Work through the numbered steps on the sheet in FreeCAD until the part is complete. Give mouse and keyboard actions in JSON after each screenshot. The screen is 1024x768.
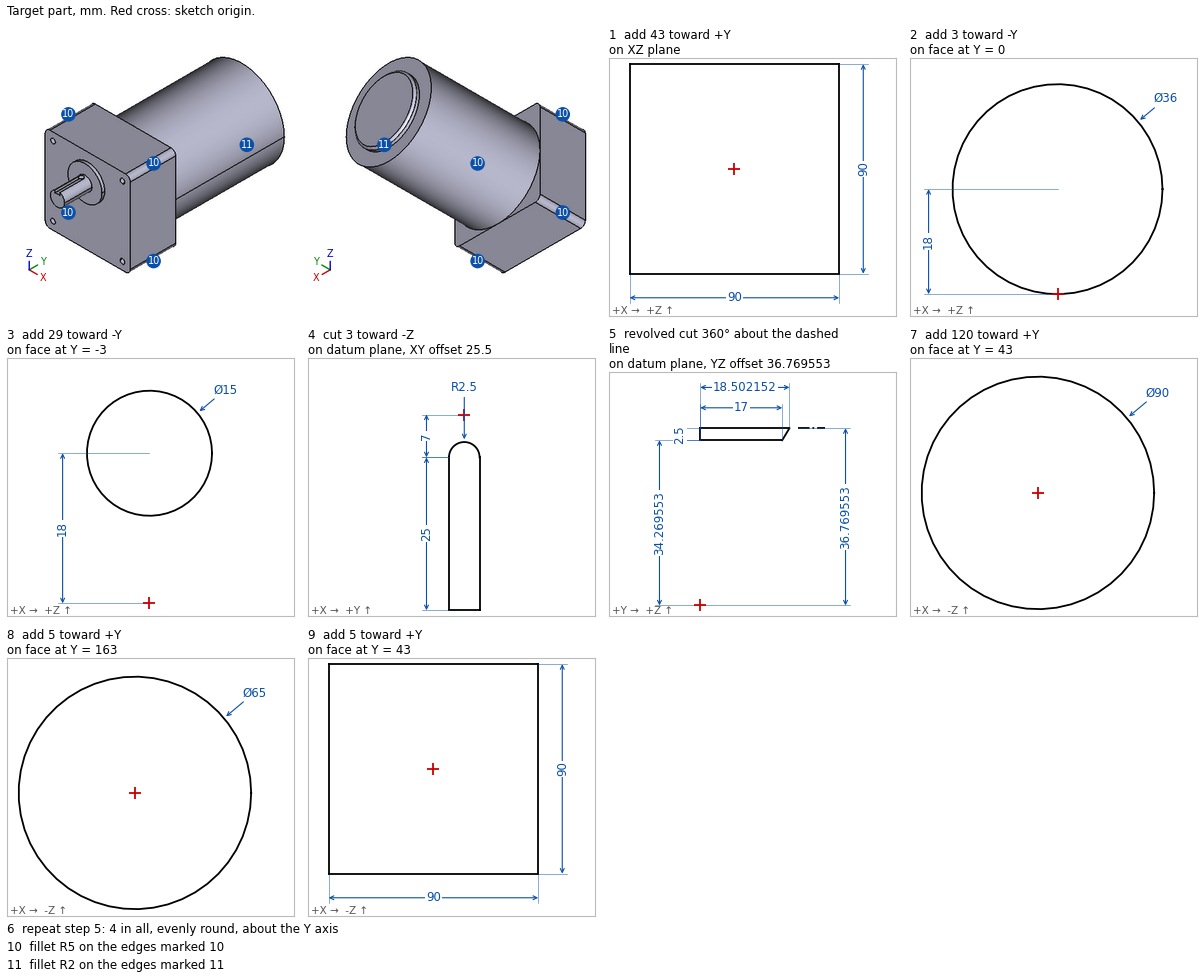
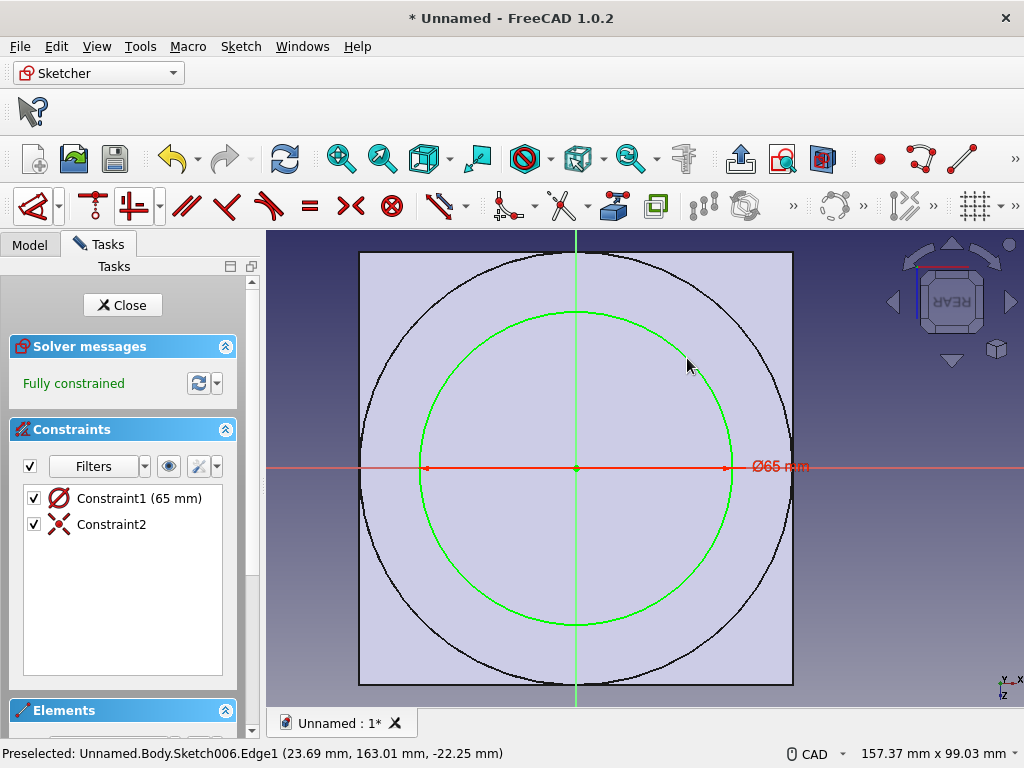
{"action": "left_click", "coordinate": [123, 305]}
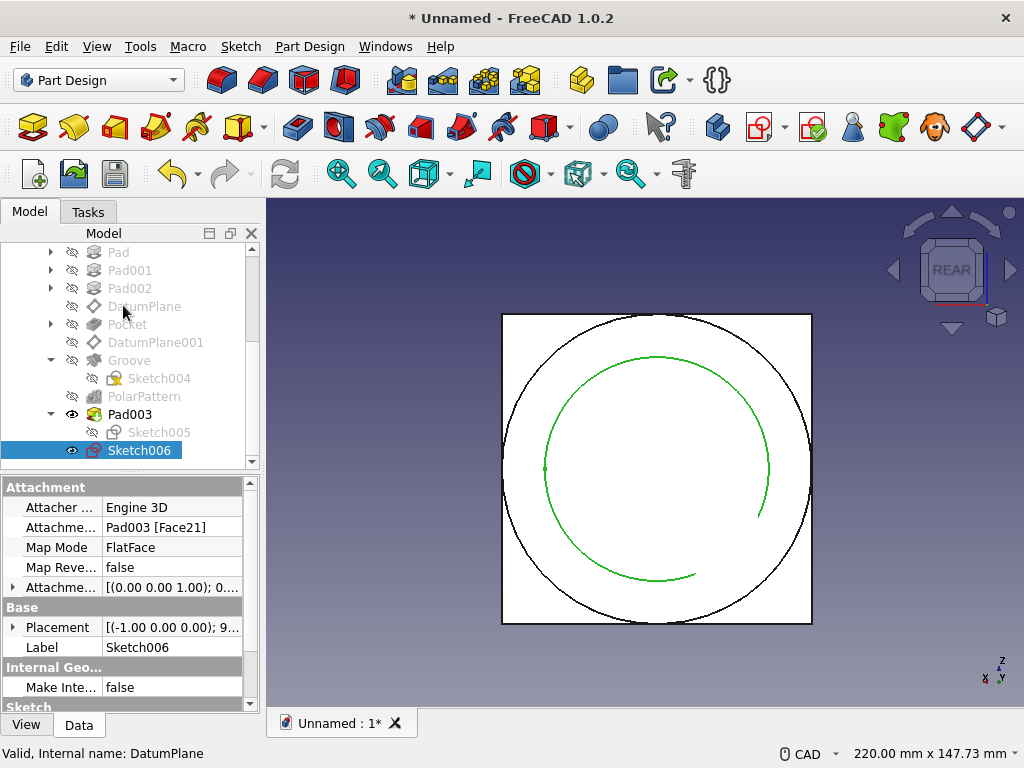
{"action": "left_click", "coordinate": [33, 128]}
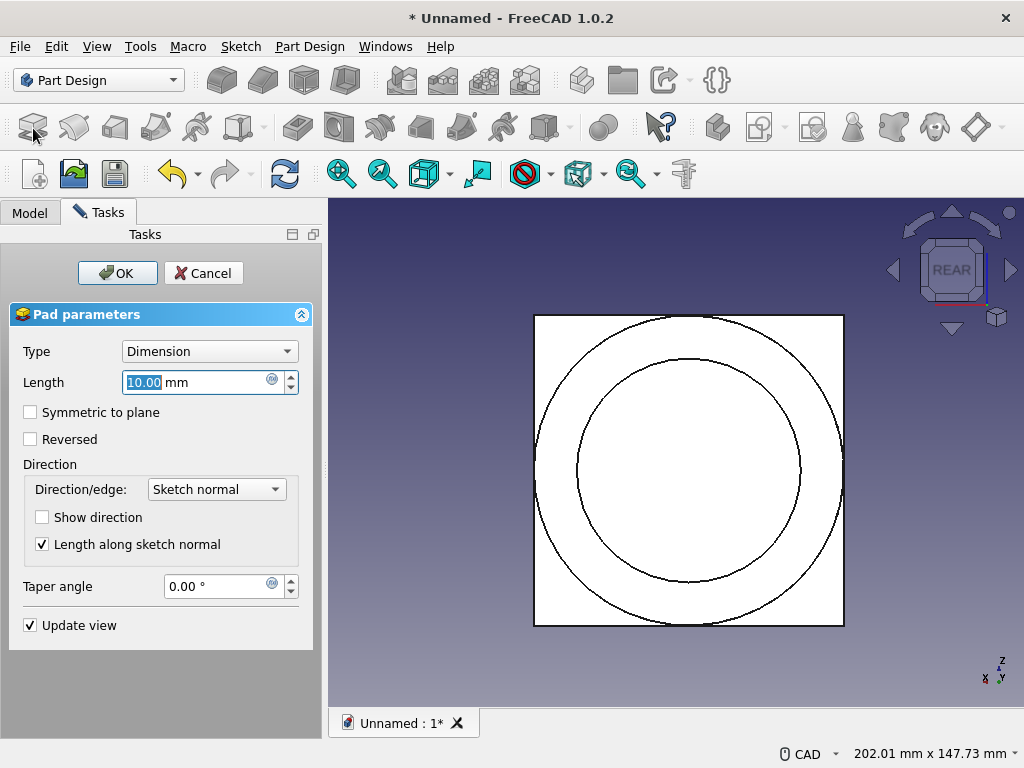
{"action": "type", "text": "5"}
{"action": "key", "text": "Tab"}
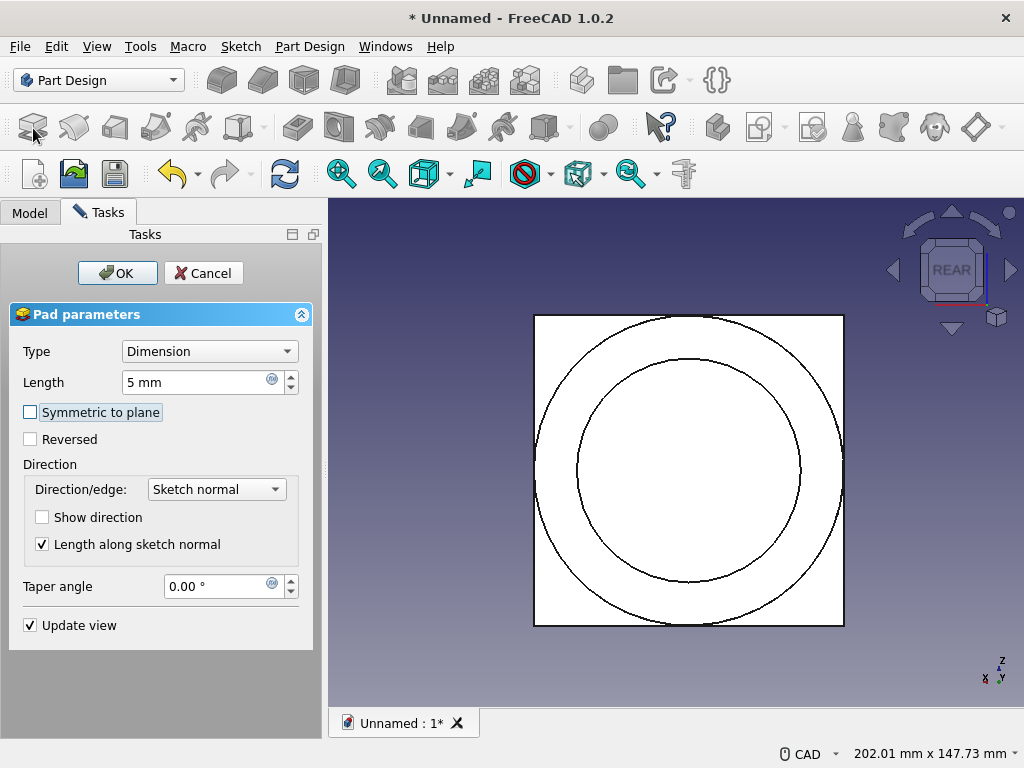
{"action": "left_click", "coordinate": [118, 273]}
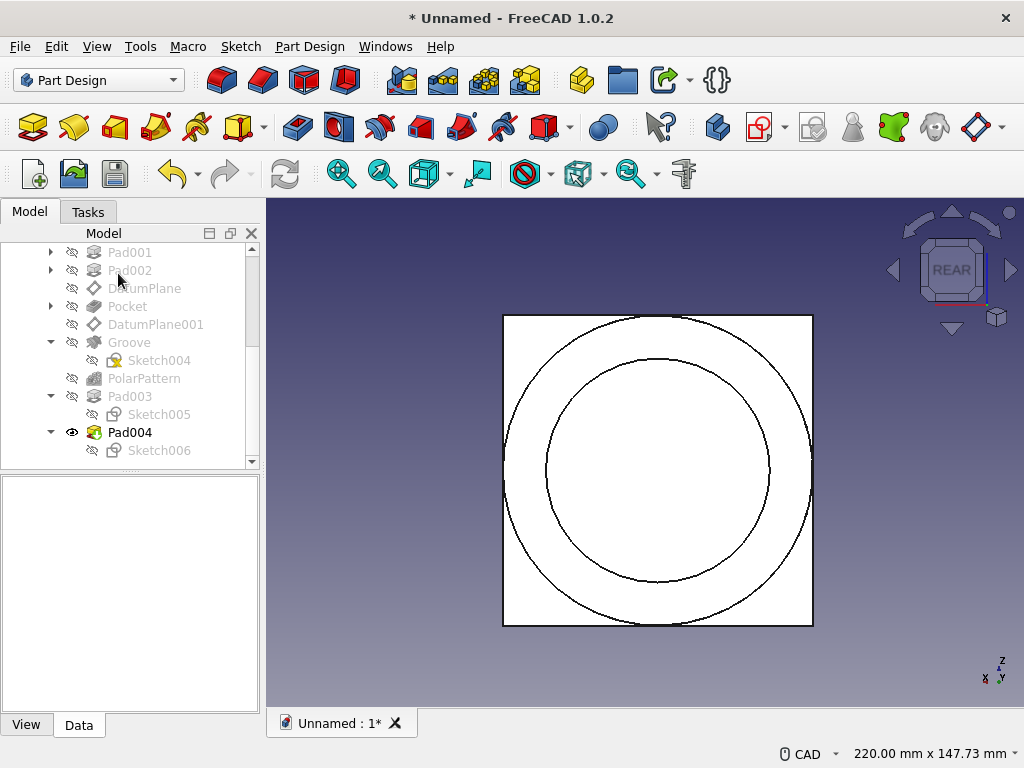
{"action": "left_click", "coordinate": [536, 348]}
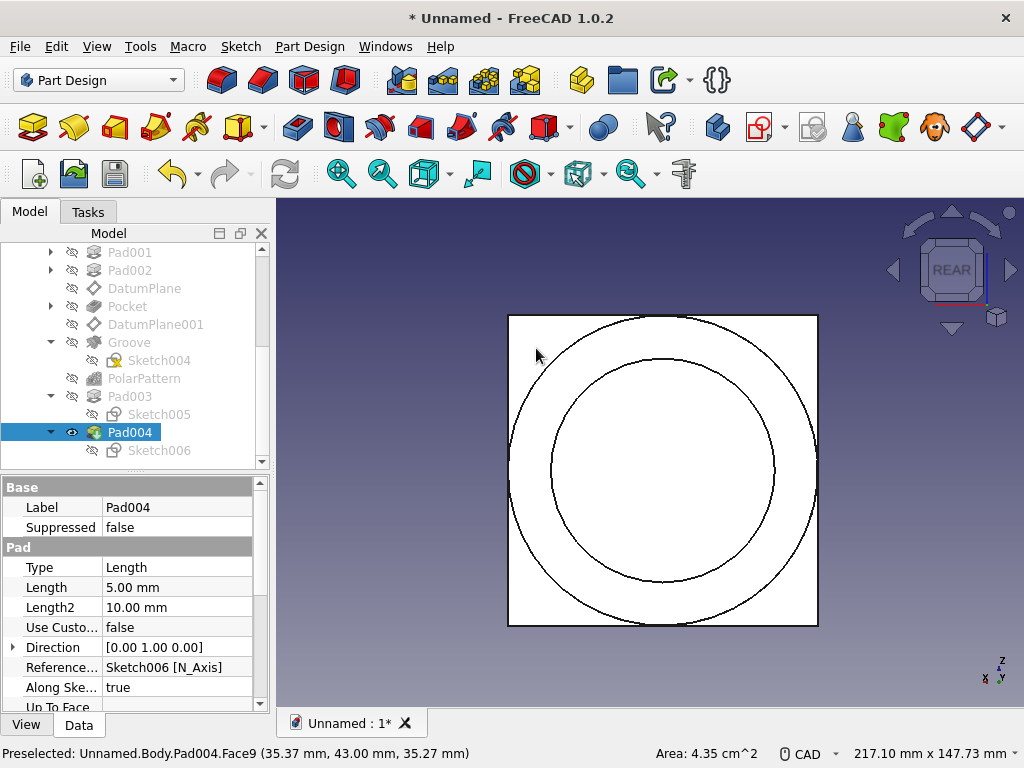
{"action": "left_click", "coordinate": [758, 128]}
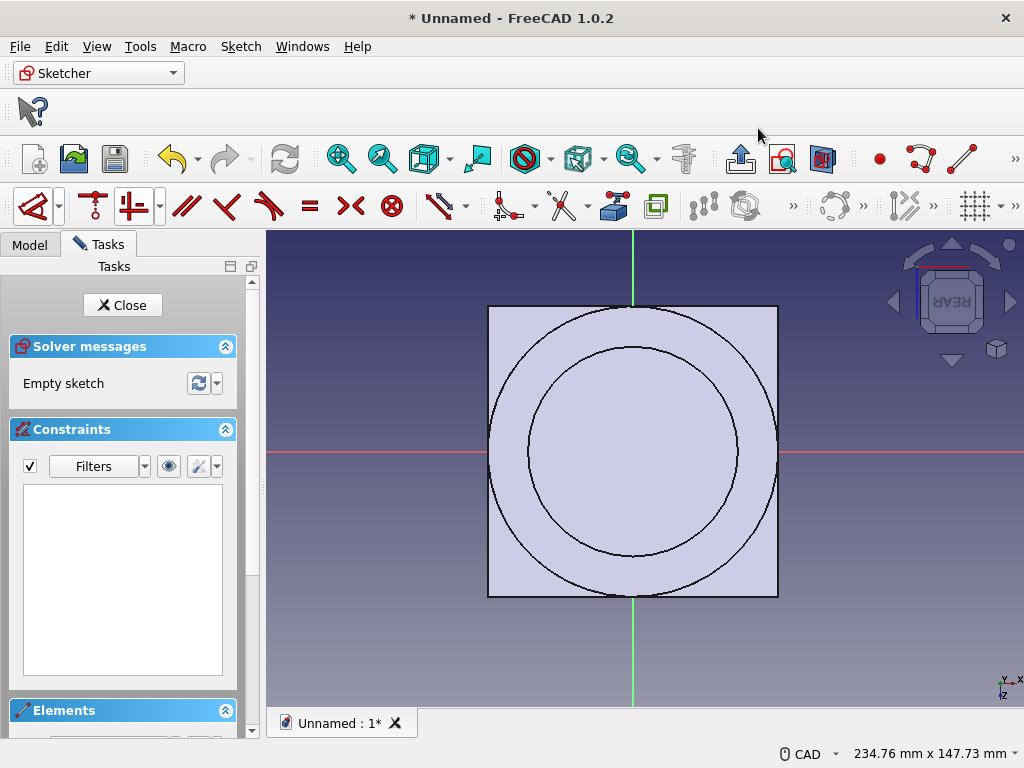
{"action": "left_click", "coordinate": [823, 160]}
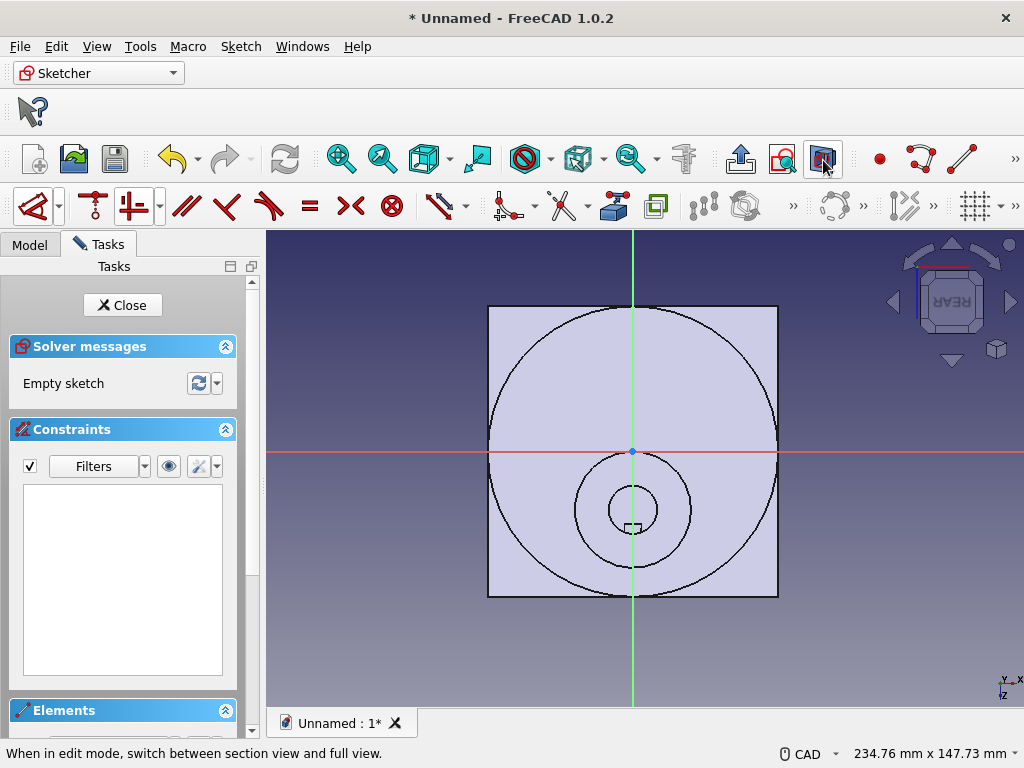
{"action": "key", "text": "g v"}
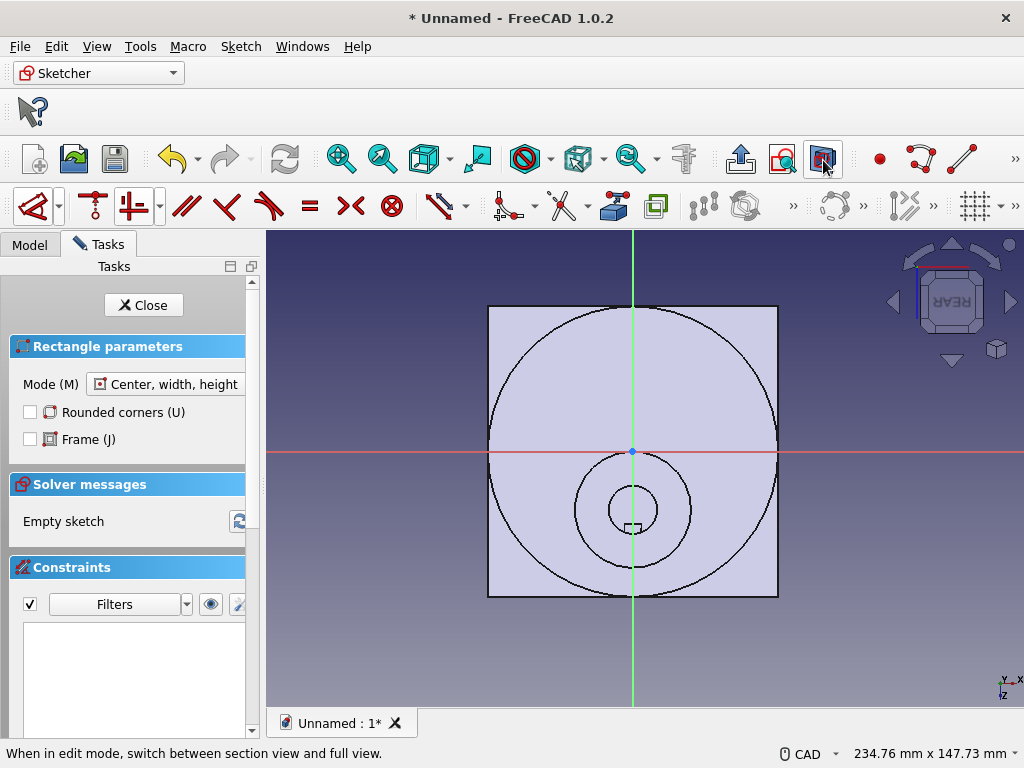
{"action": "left_click", "coordinate": [633, 452]}
{"action": "mouse_move", "coordinate": [778, 306]}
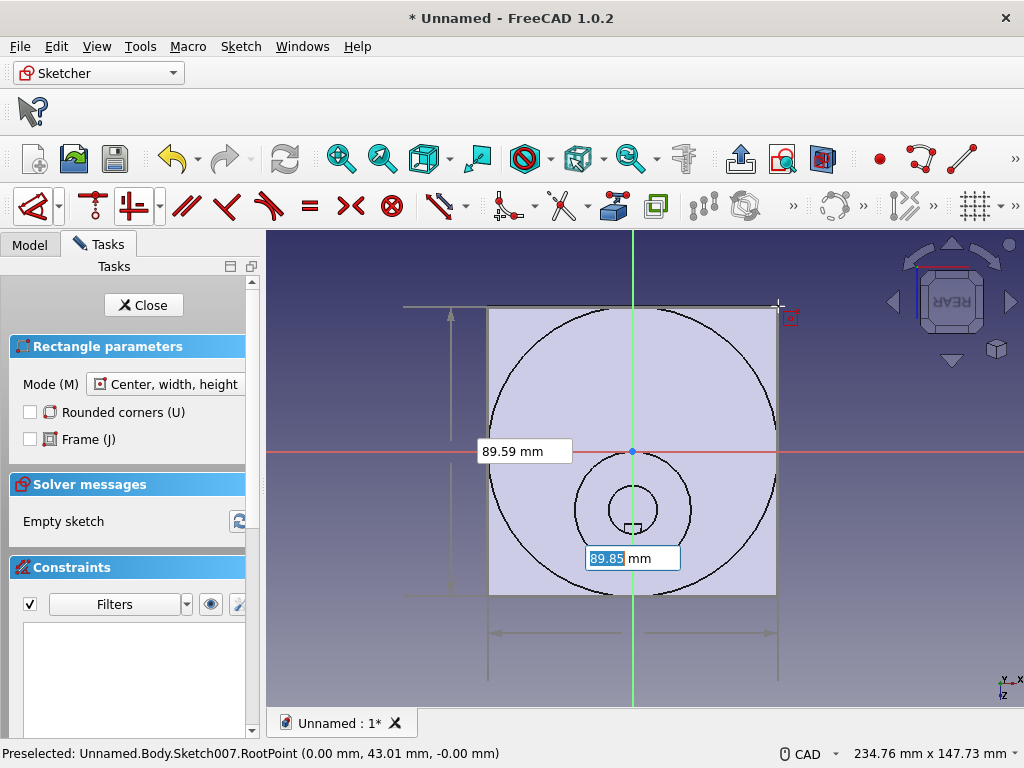
{"action": "type", "text": "90"}
{"action": "key", "text": "Tab"}
{"action": "type", "text": "90"}
{"action": "key", "text": "Return"}
{"action": "key", "text": "Escape"}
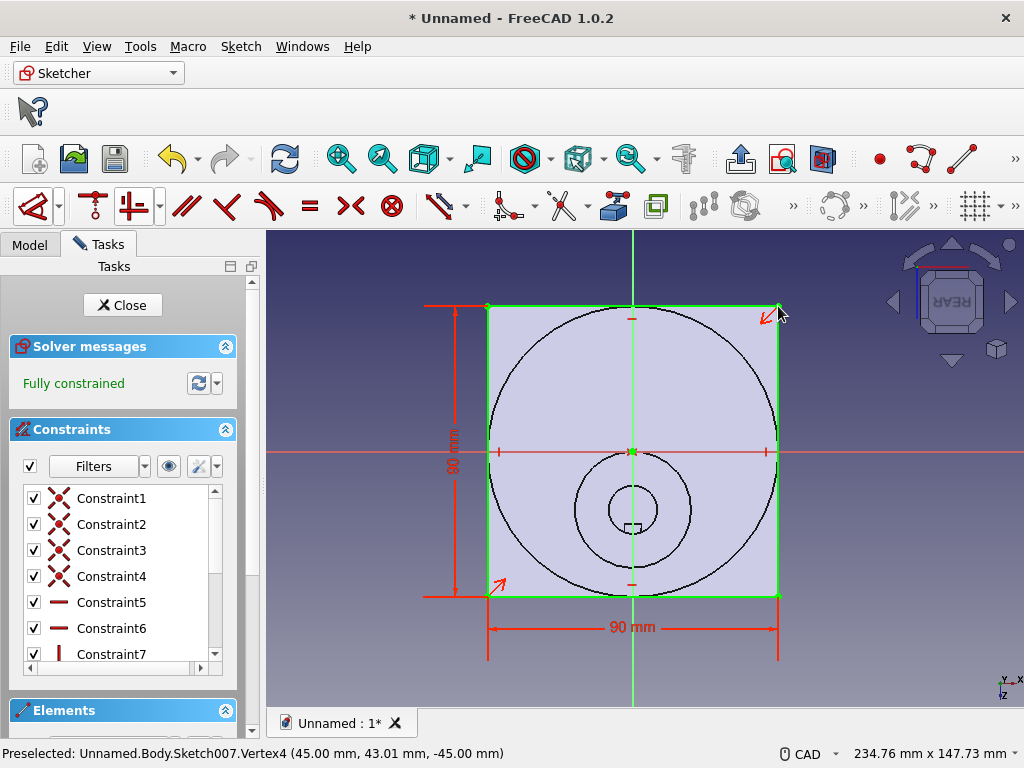
{"action": "left_click", "coordinate": [123, 305]}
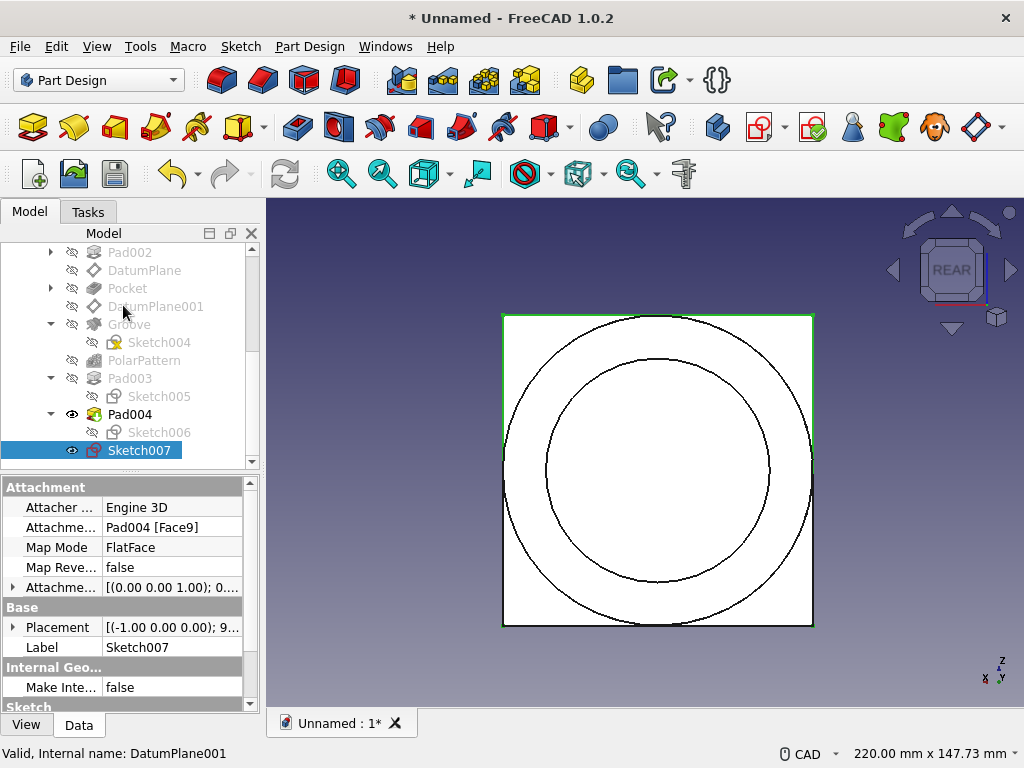
{"action": "left_click", "coordinate": [33, 128]}